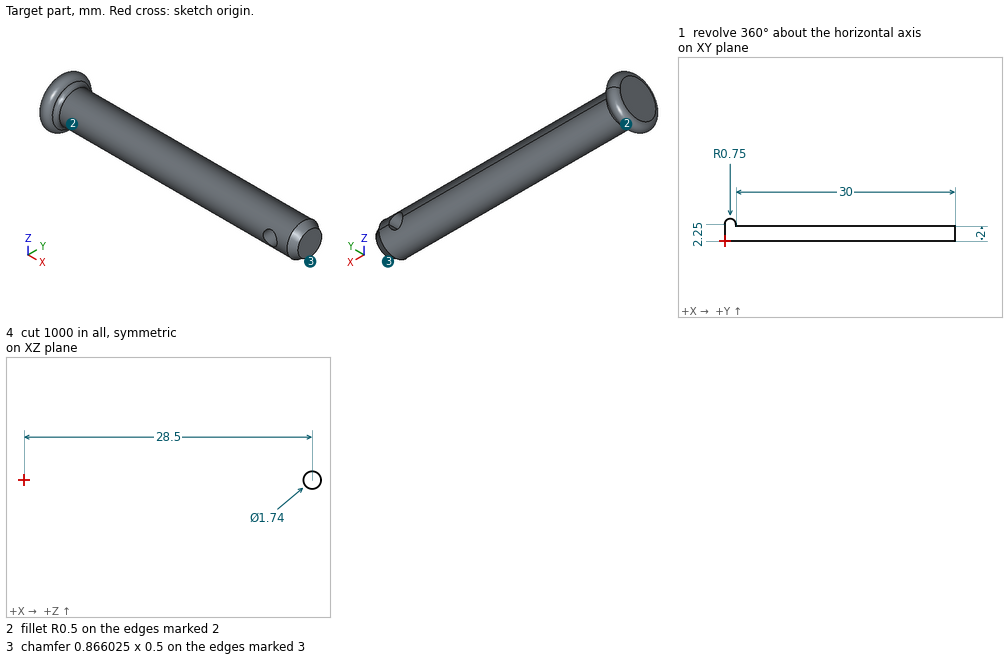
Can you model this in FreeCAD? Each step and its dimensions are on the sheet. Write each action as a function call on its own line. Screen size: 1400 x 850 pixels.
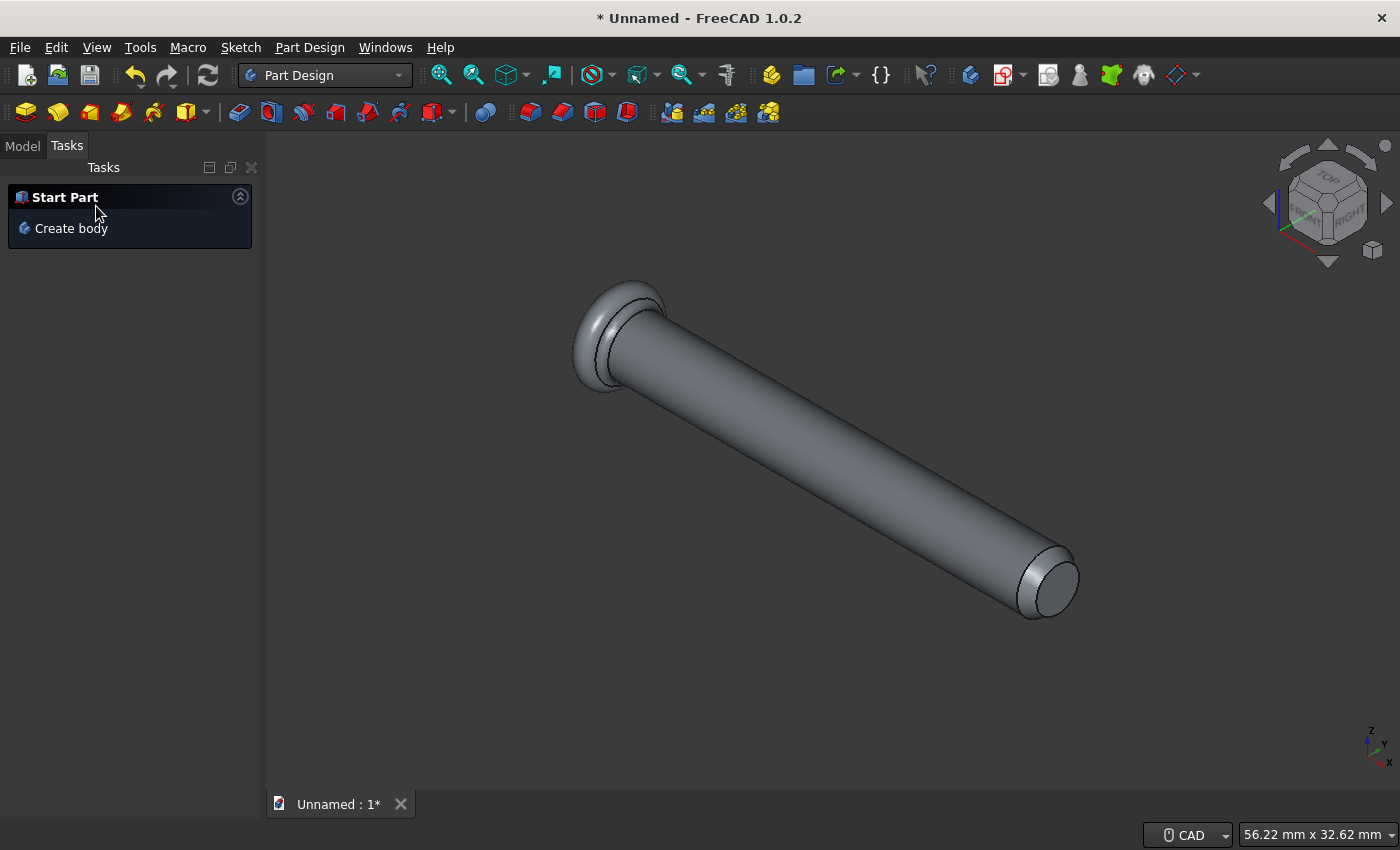
click(1004, 76)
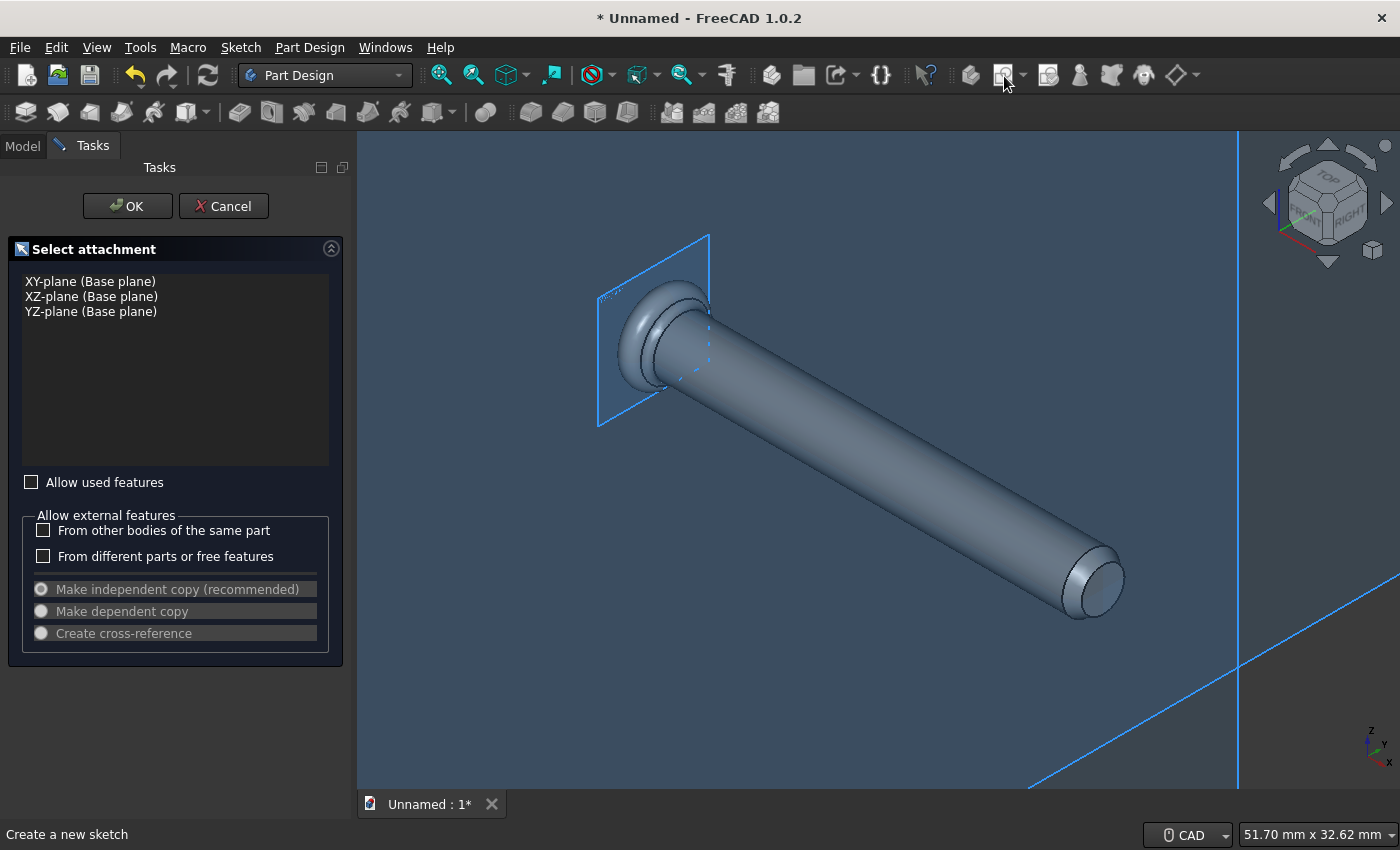
click(82, 296)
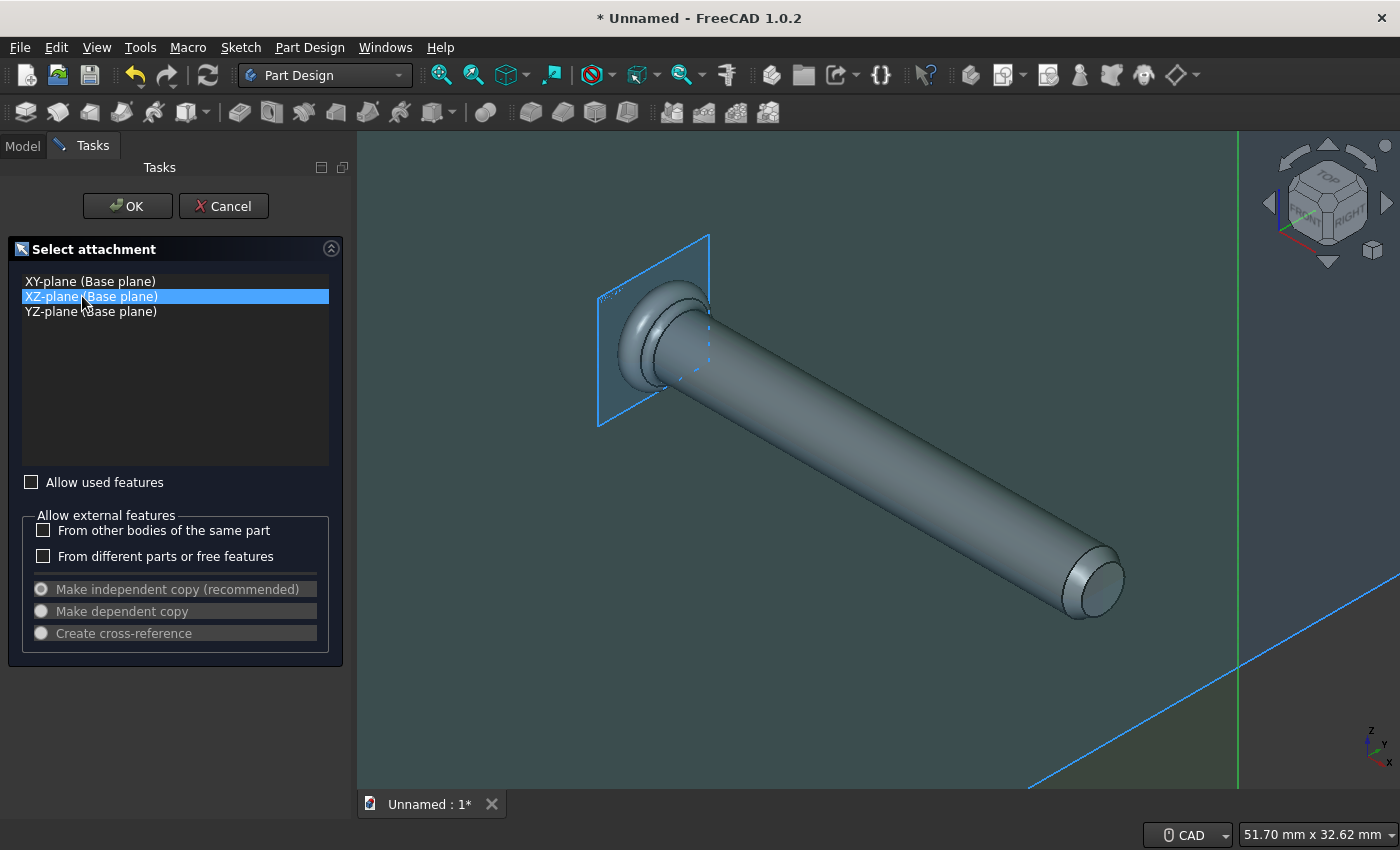
click(128, 206)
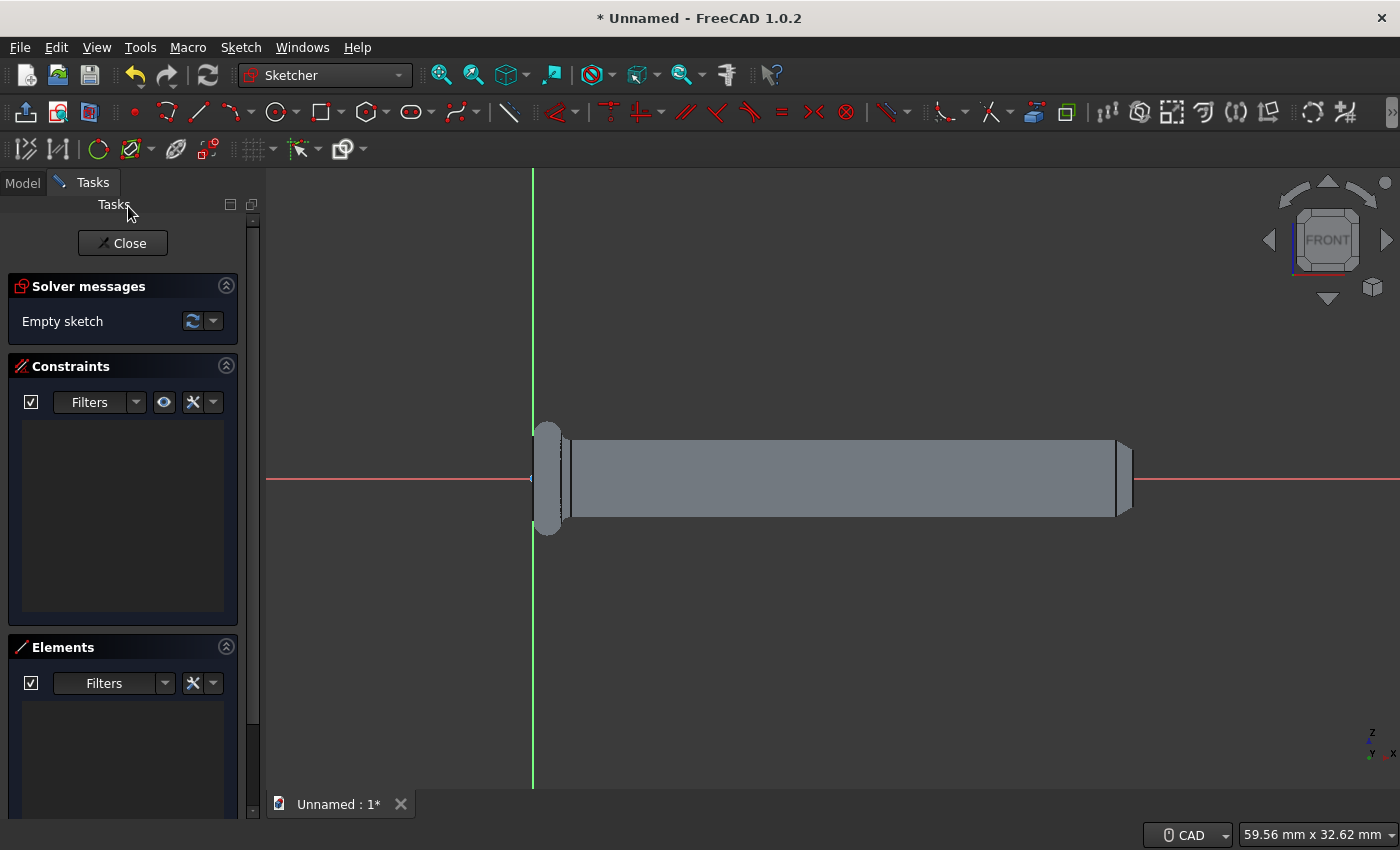
click(90, 112)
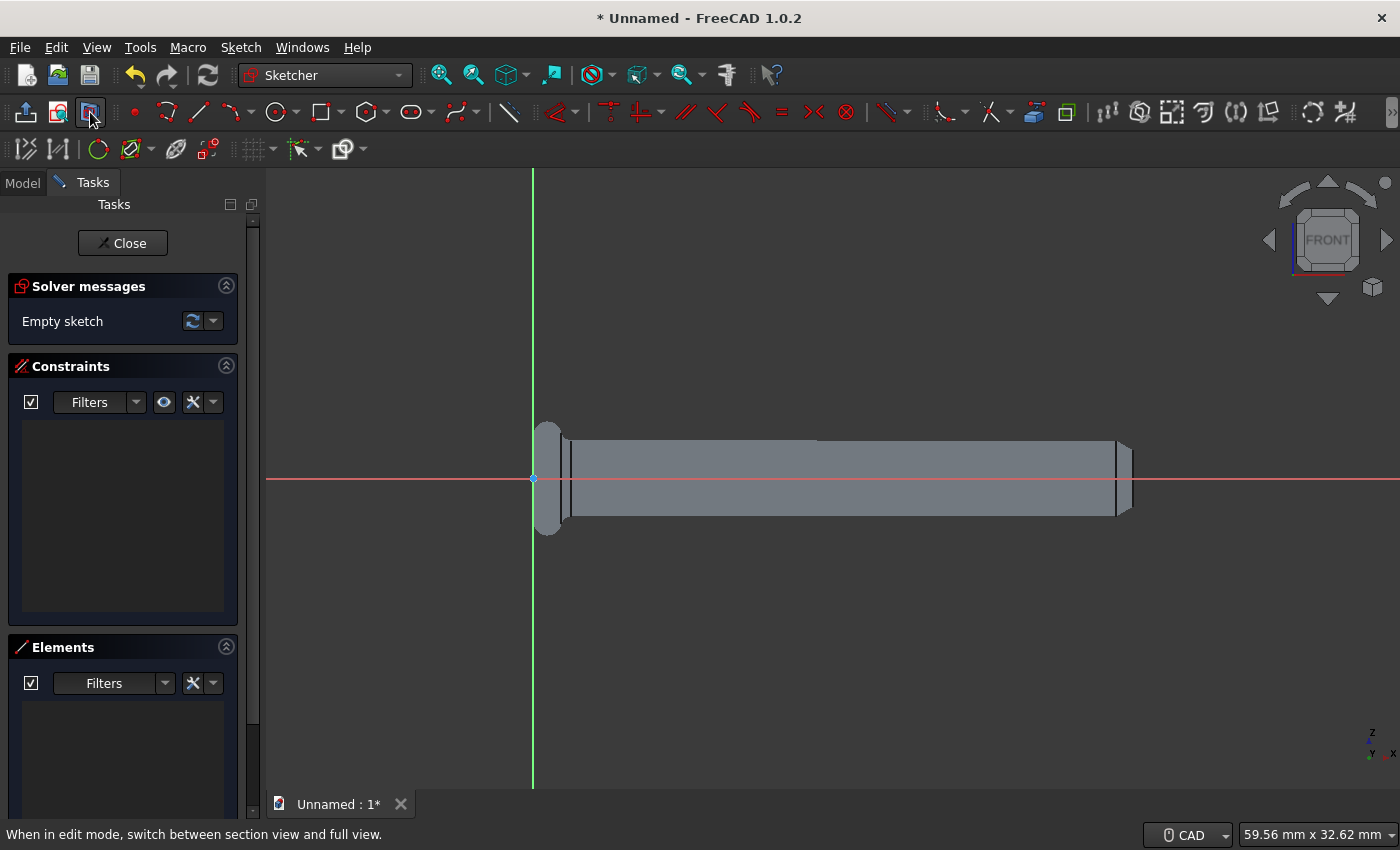
scroll(1107, 478, up, 12)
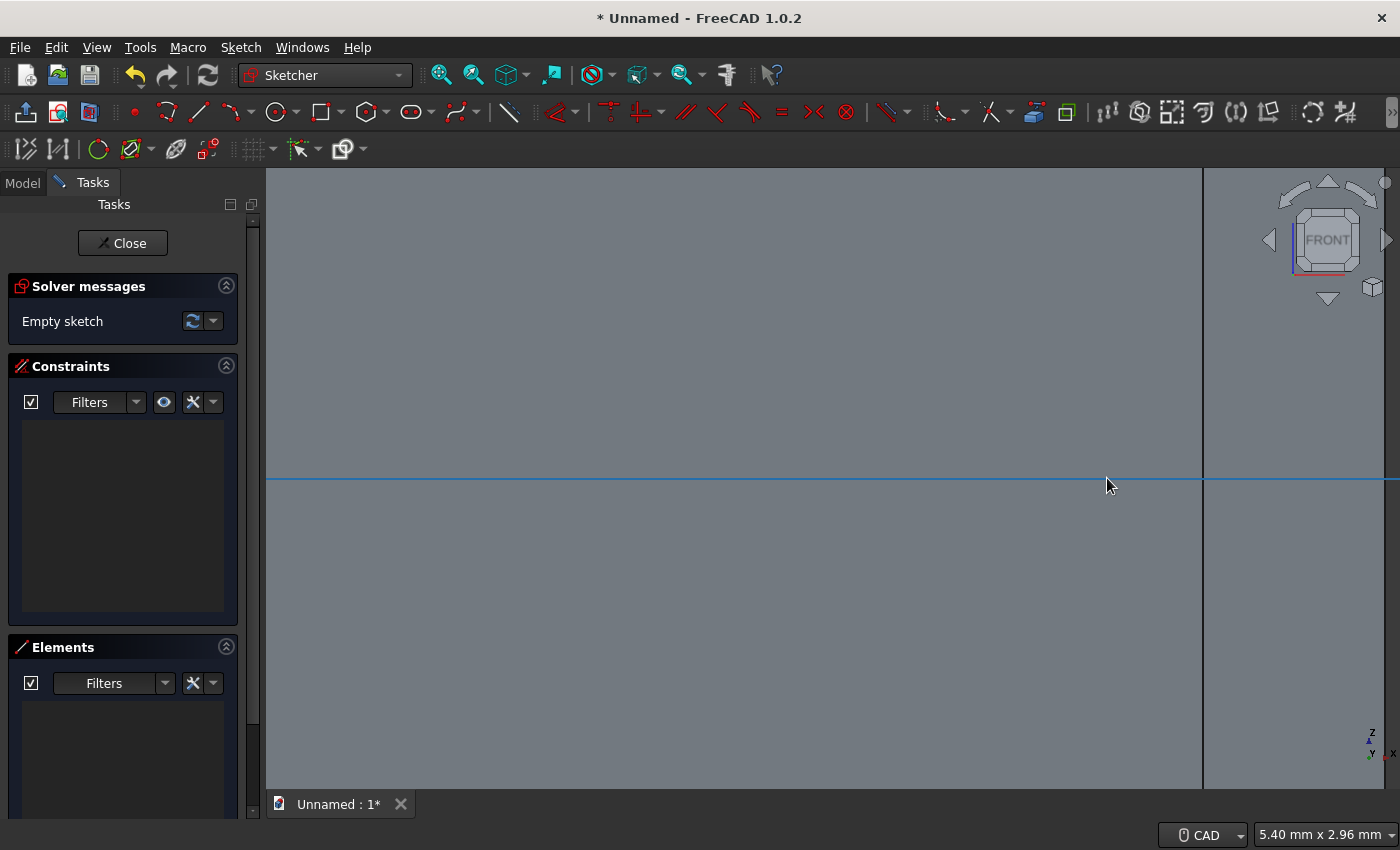
click(276, 112)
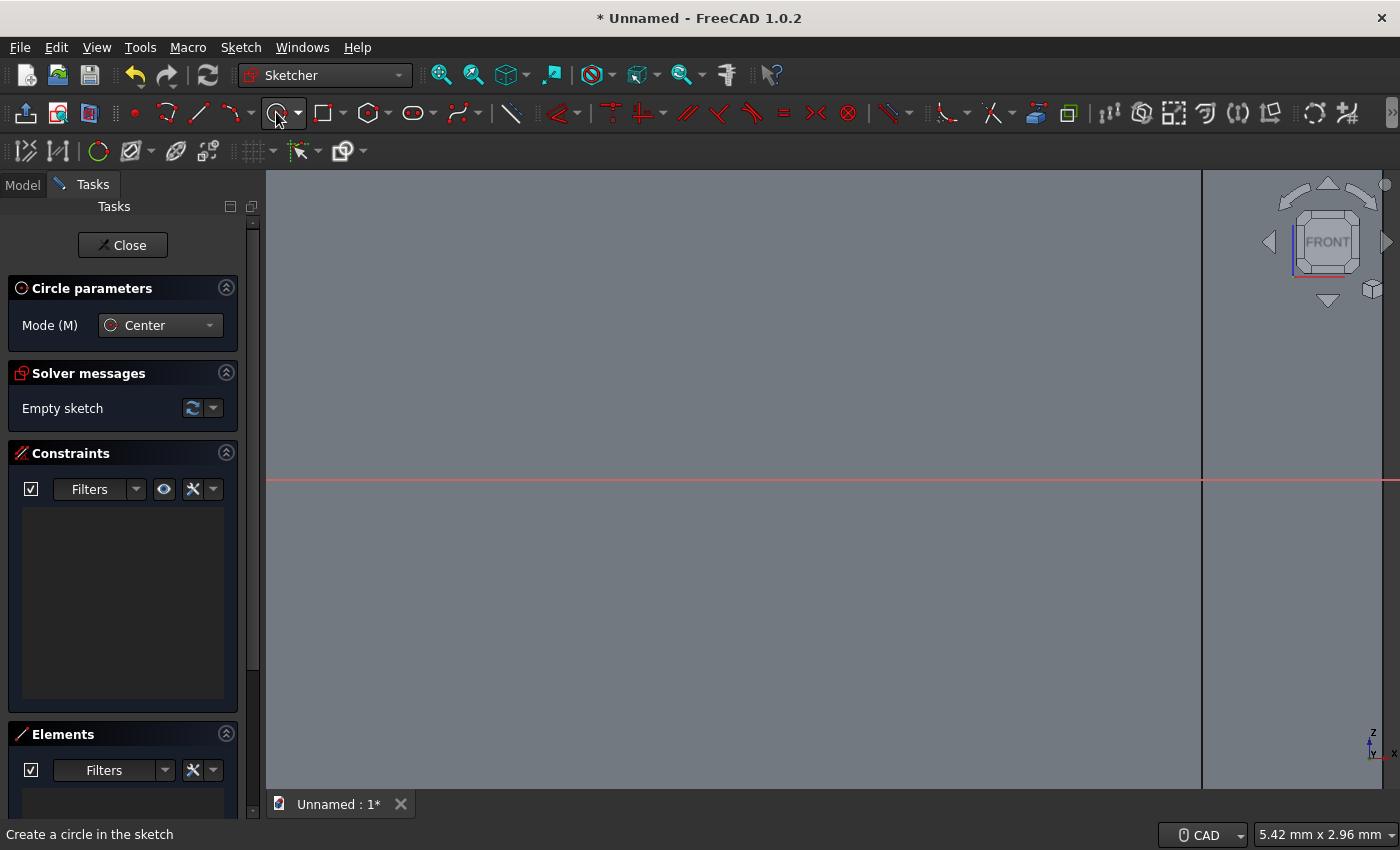
click(755, 479)
click(884, 351)
key(Escape)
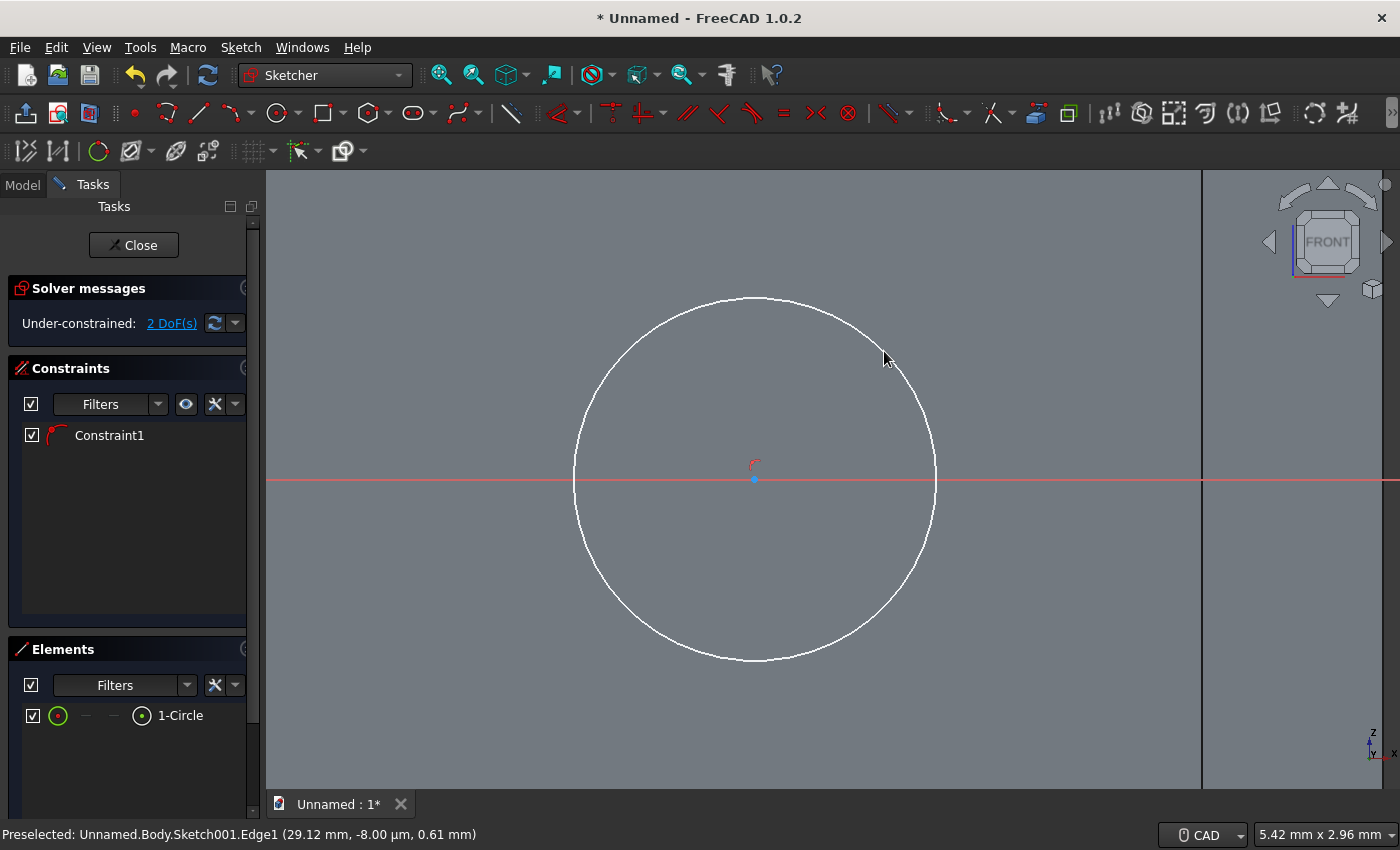
click(558, 114)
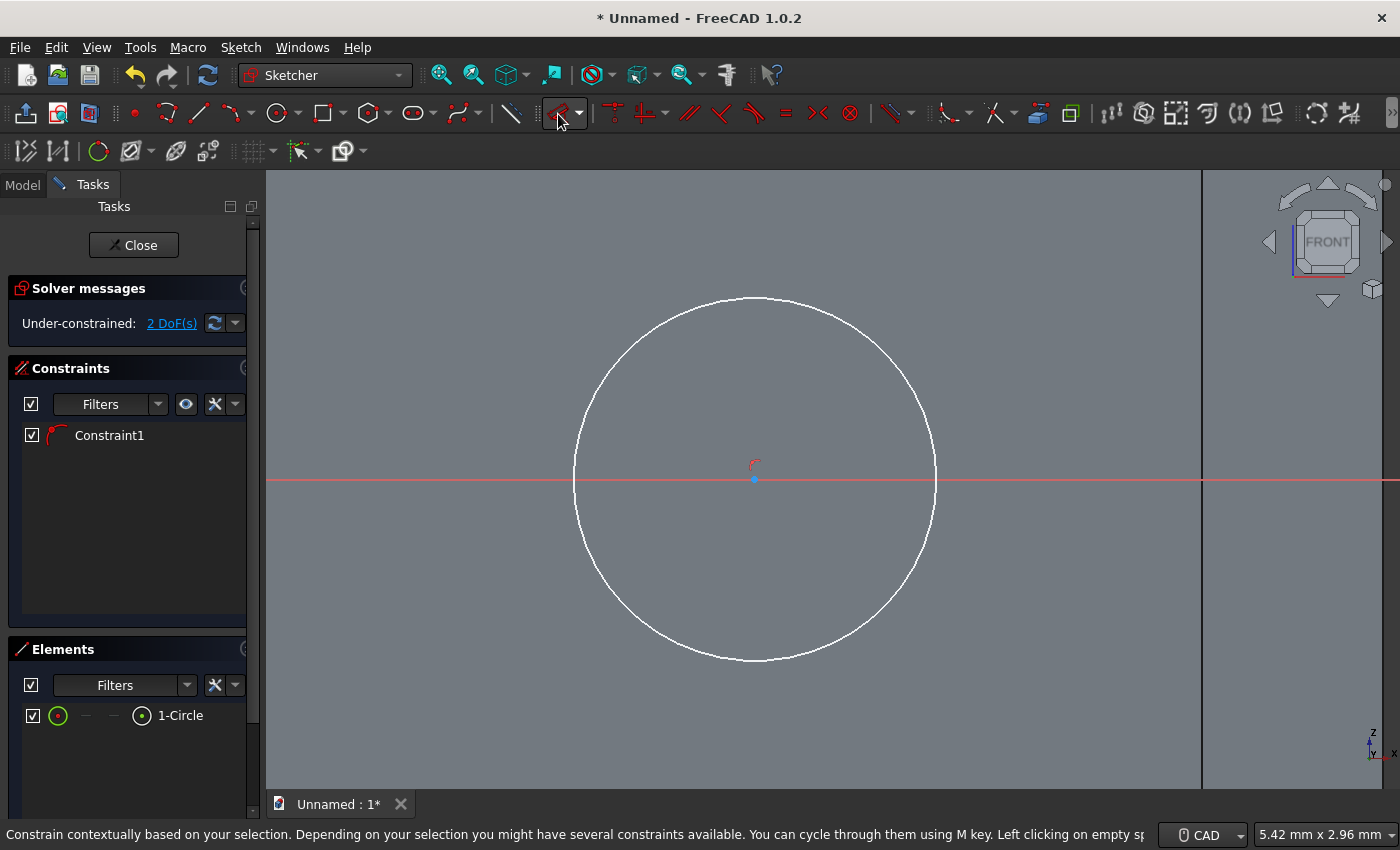
click(883, 351)
click(906, 328)